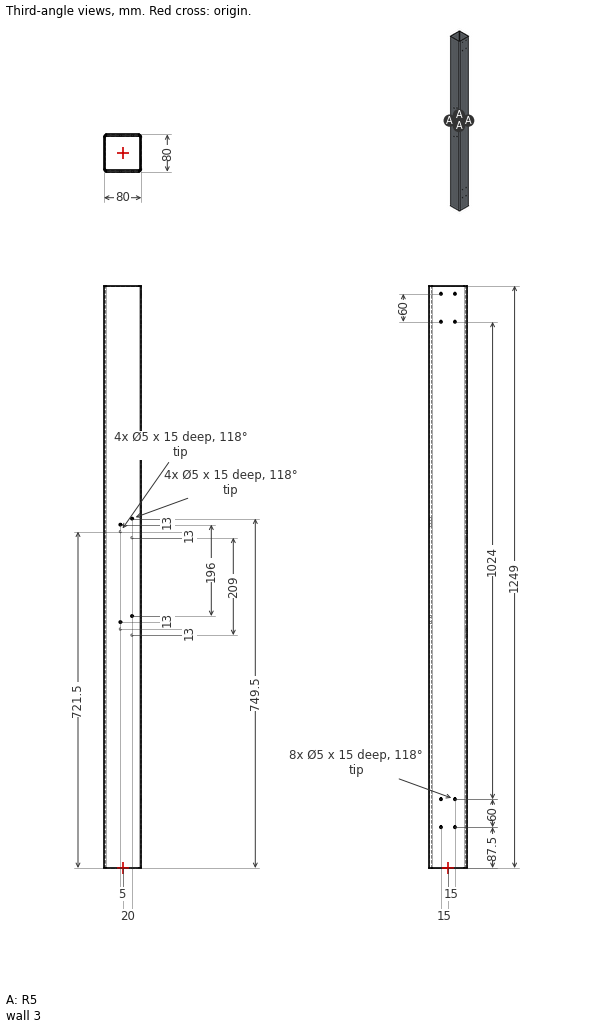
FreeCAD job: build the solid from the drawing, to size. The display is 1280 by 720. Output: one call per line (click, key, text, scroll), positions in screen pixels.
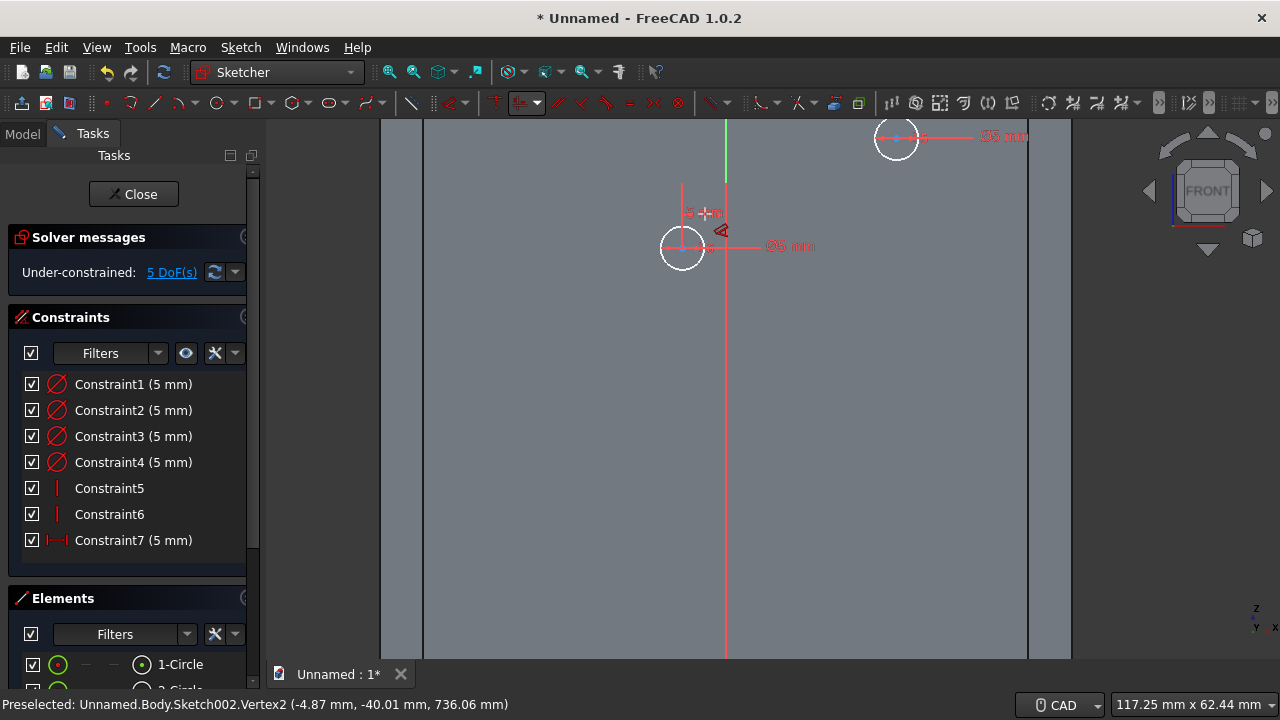
scroll(687, 250, down, 9)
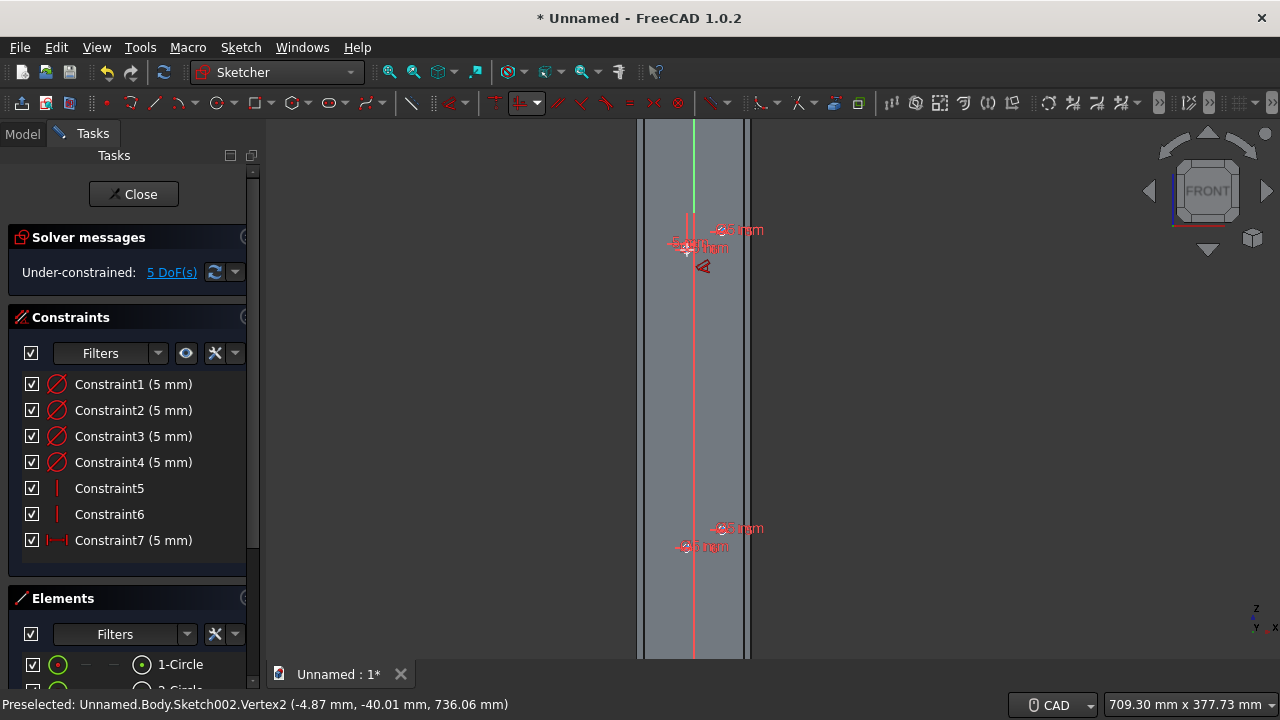
scroll(722, 232, up, 2)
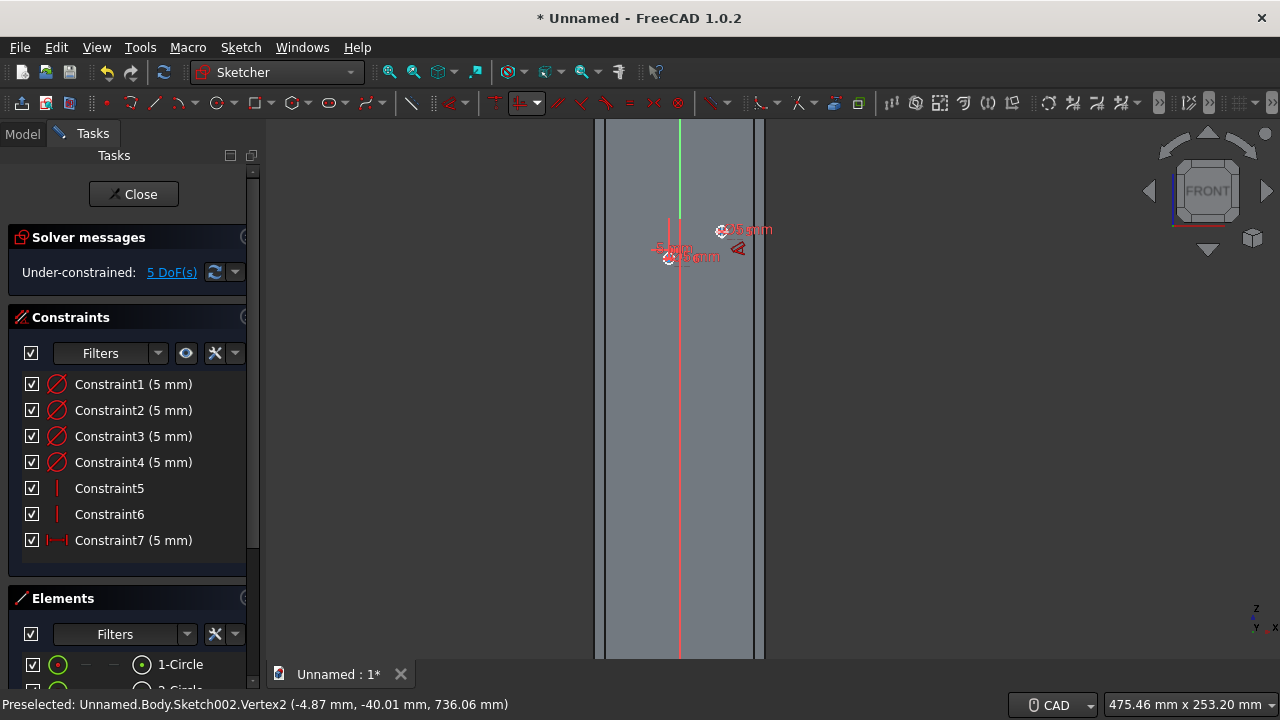
click(722, 232)
click(701, 198)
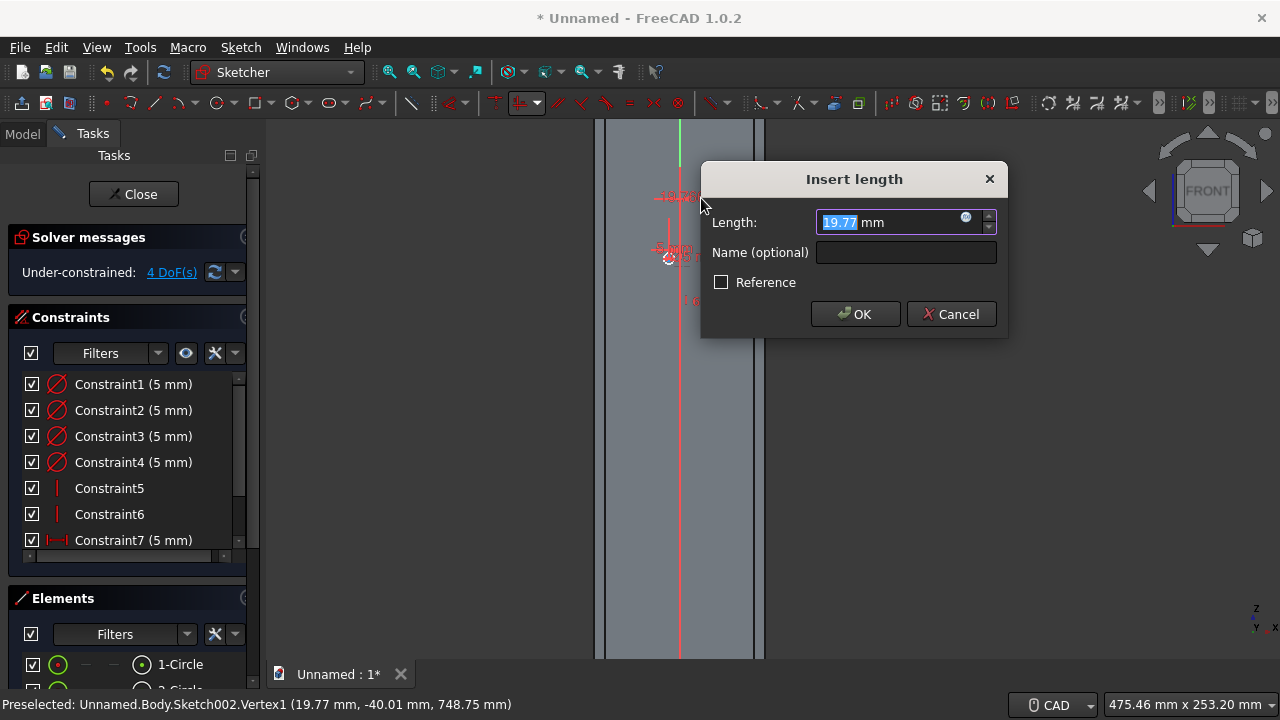
text(20)
key(Return)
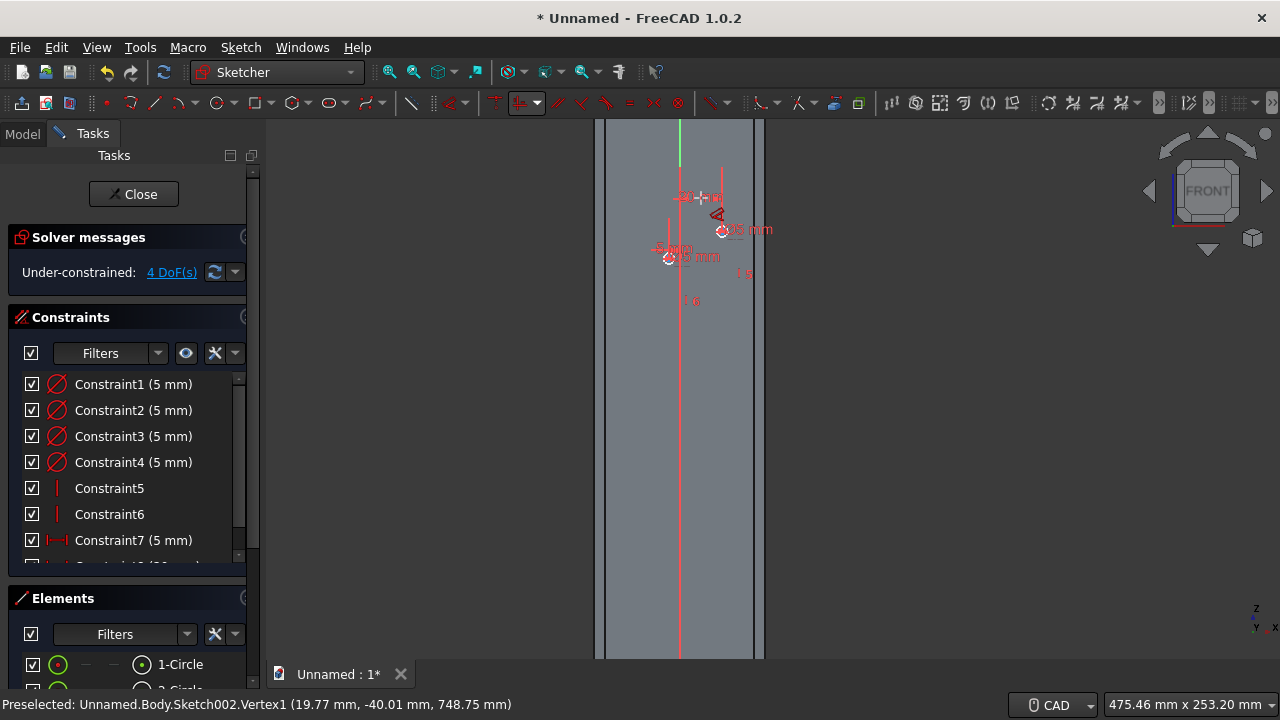
scroll(722, 232, up, 2)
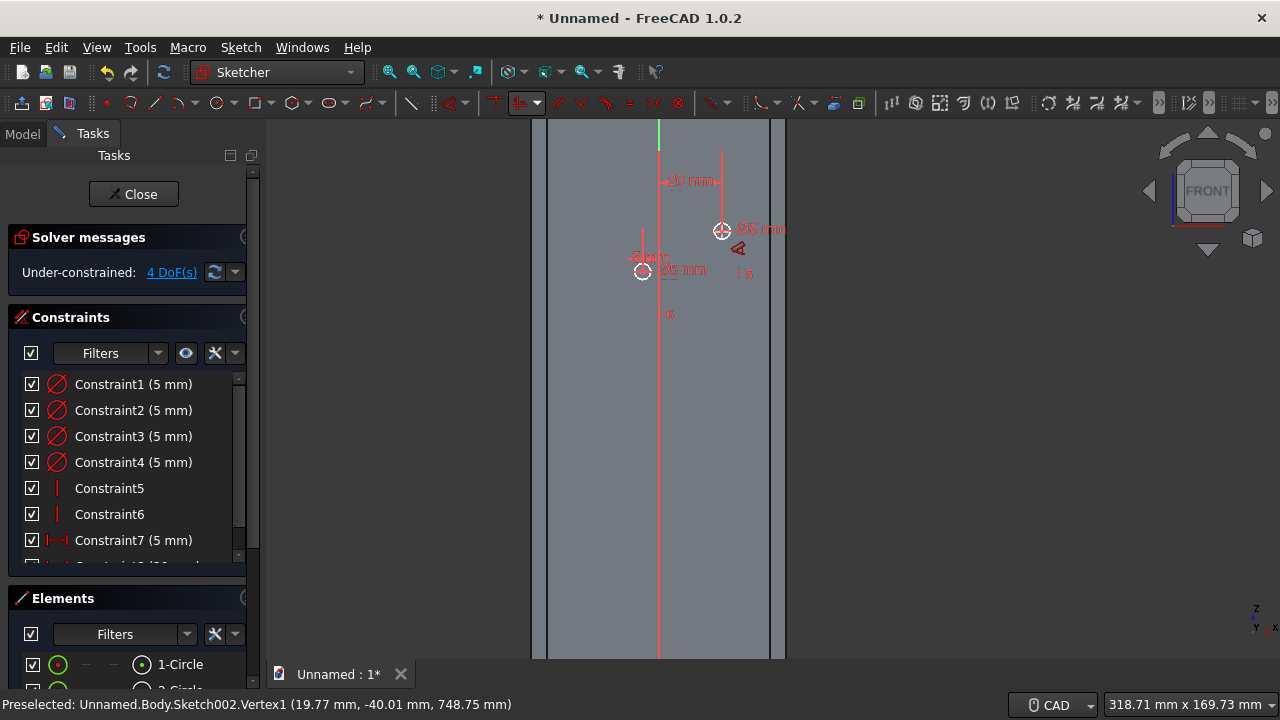
click(722, 231)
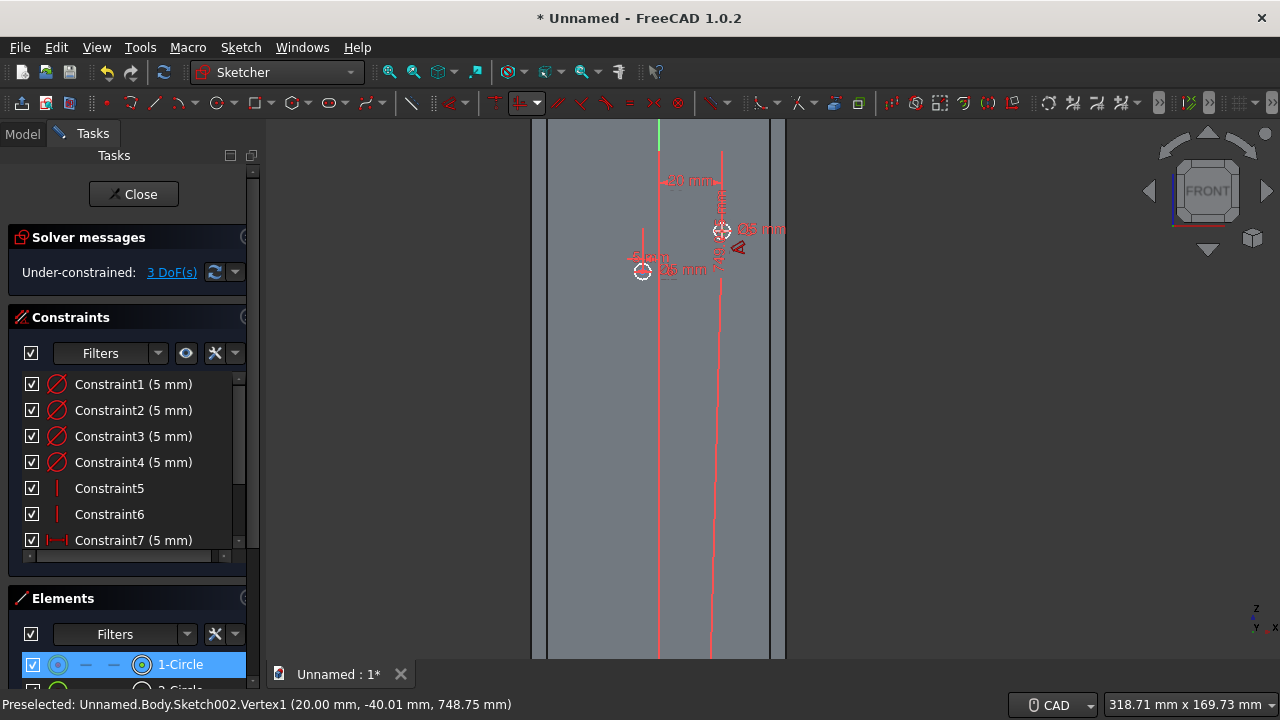
click(643, 272)
click(756, 251)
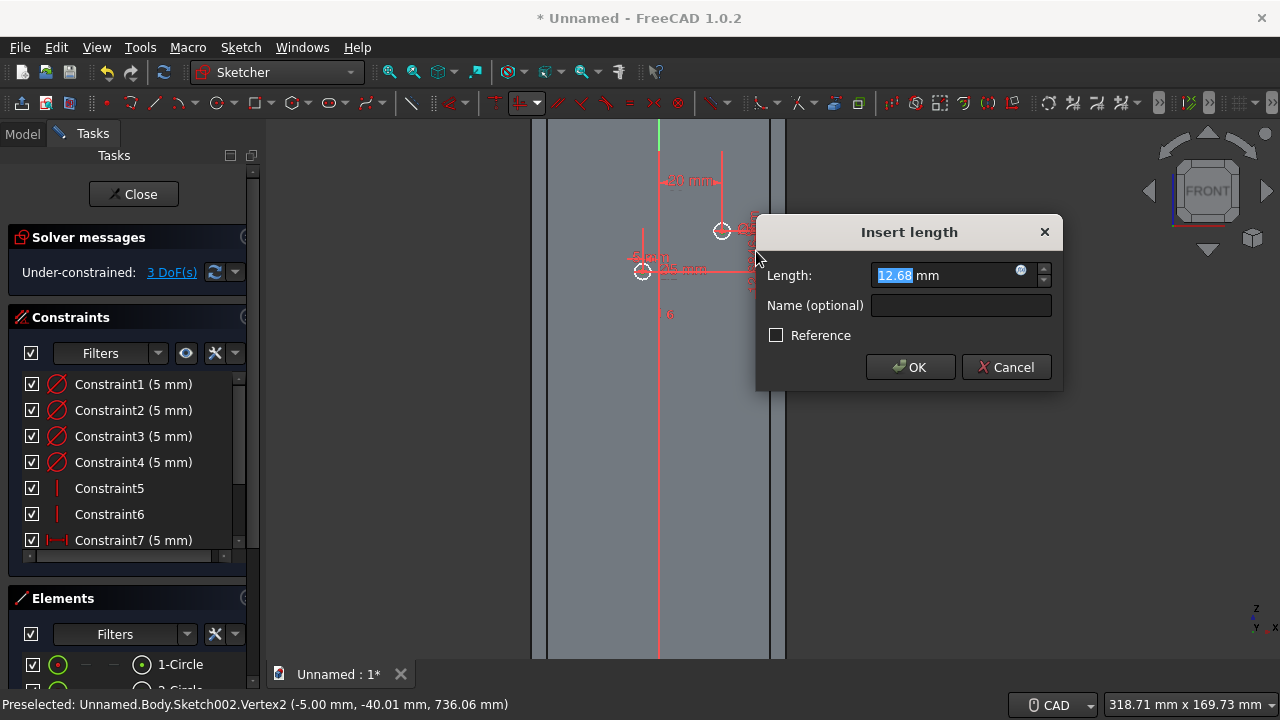
text(13)
key(Return)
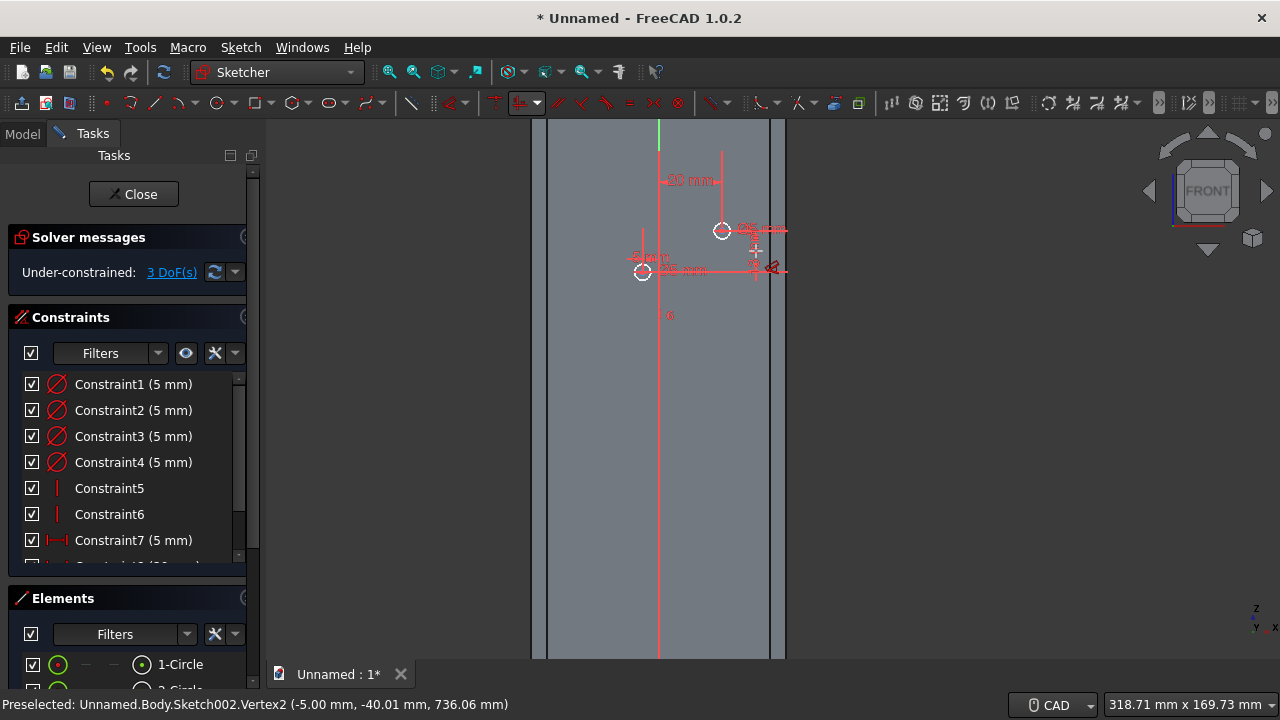
scroll(723, 232, down, 4)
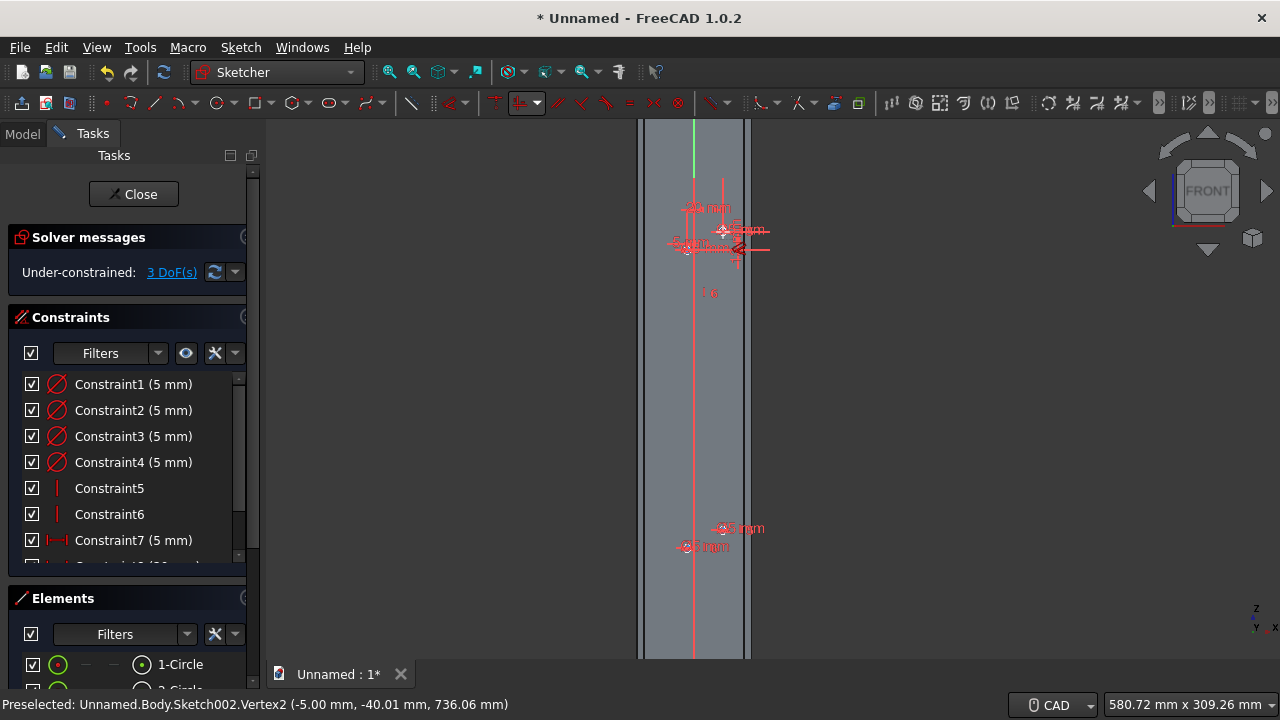
scroll(723, 530, up, 4)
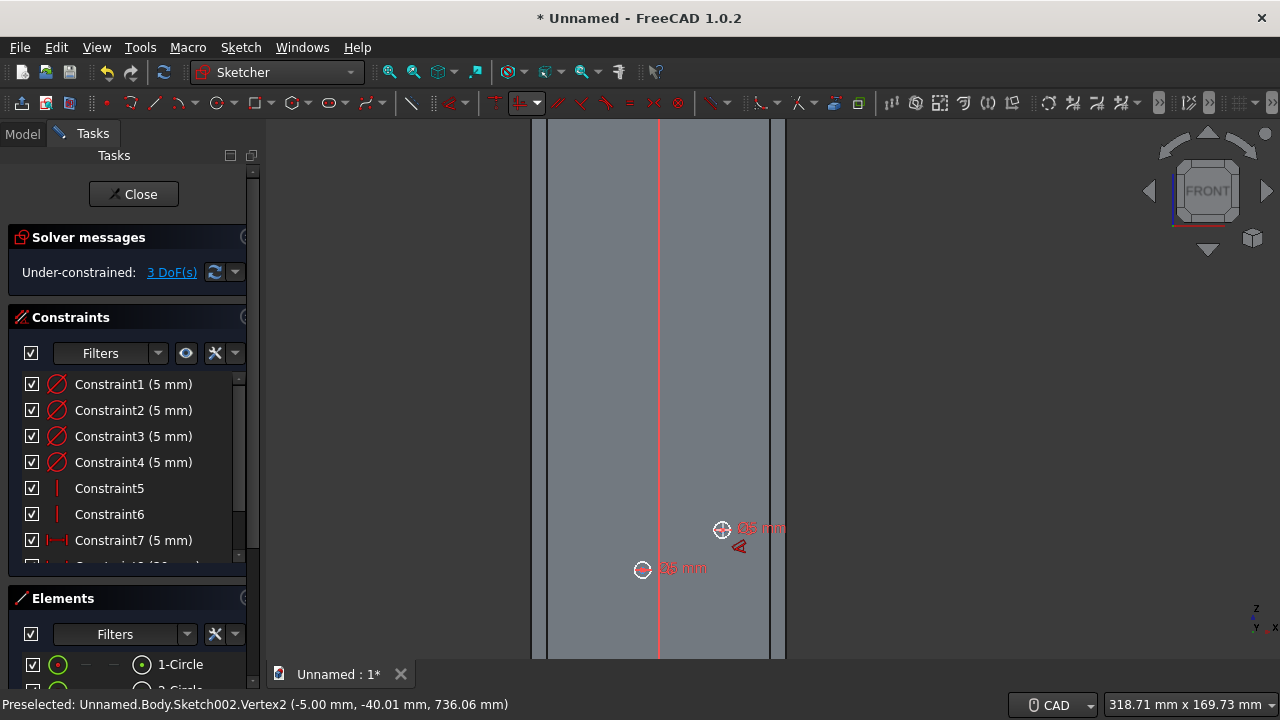
click(722, 530)